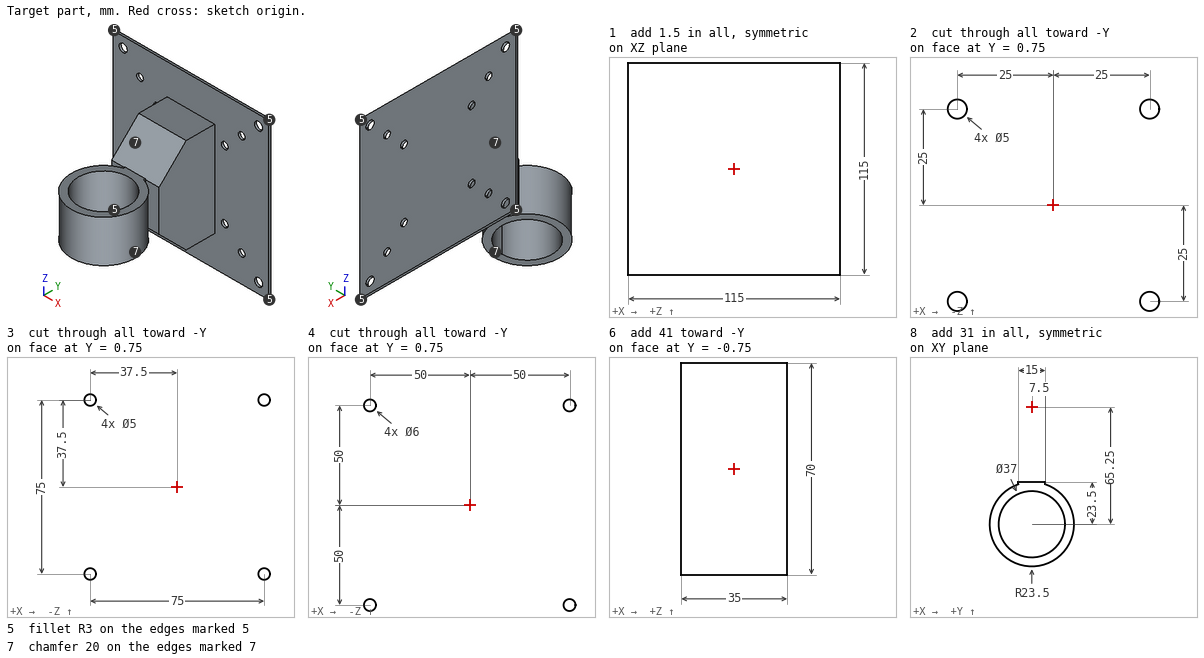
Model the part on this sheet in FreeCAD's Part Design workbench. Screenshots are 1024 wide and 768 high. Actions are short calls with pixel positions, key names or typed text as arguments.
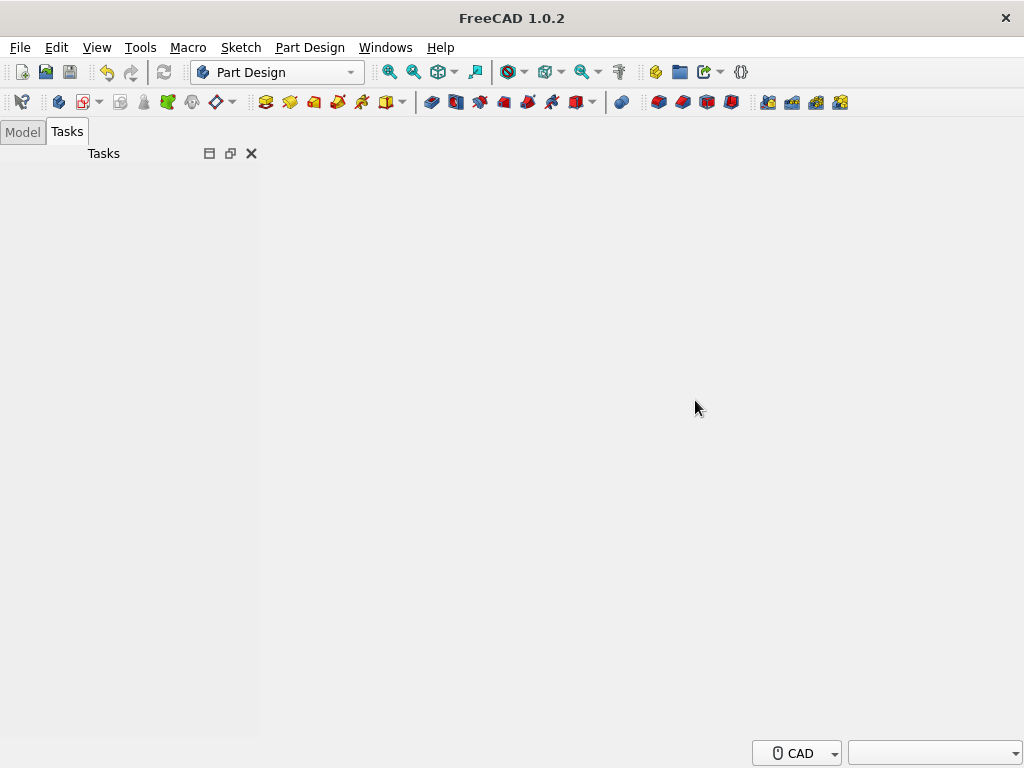
click(22, 72)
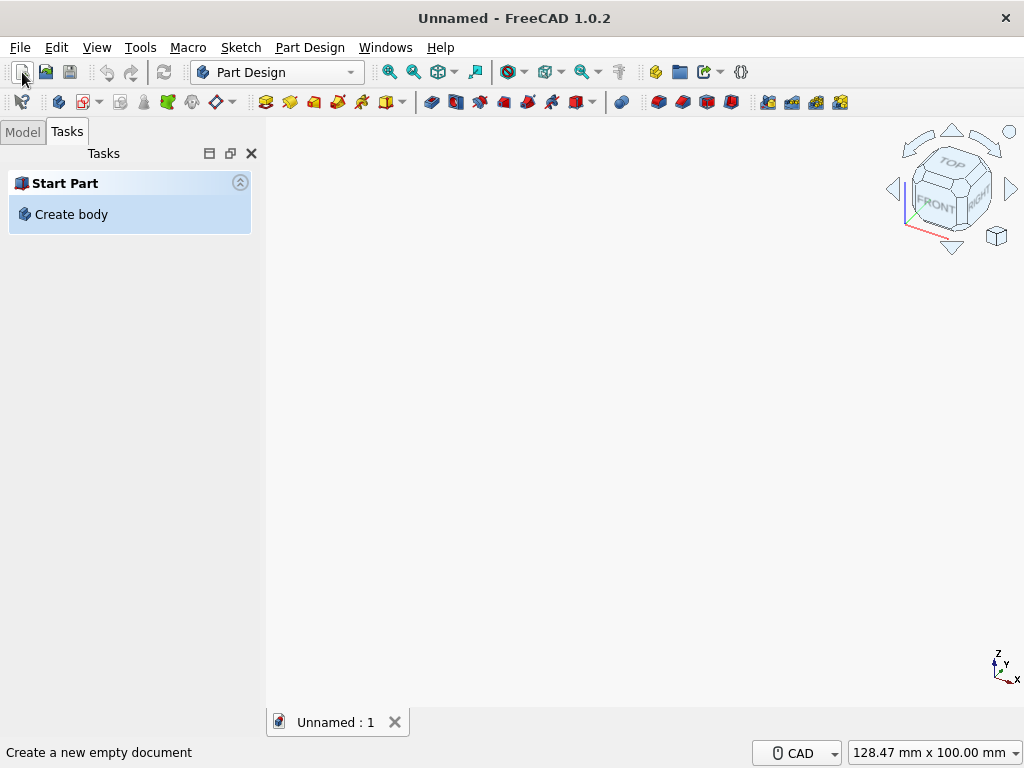
click(84, 102)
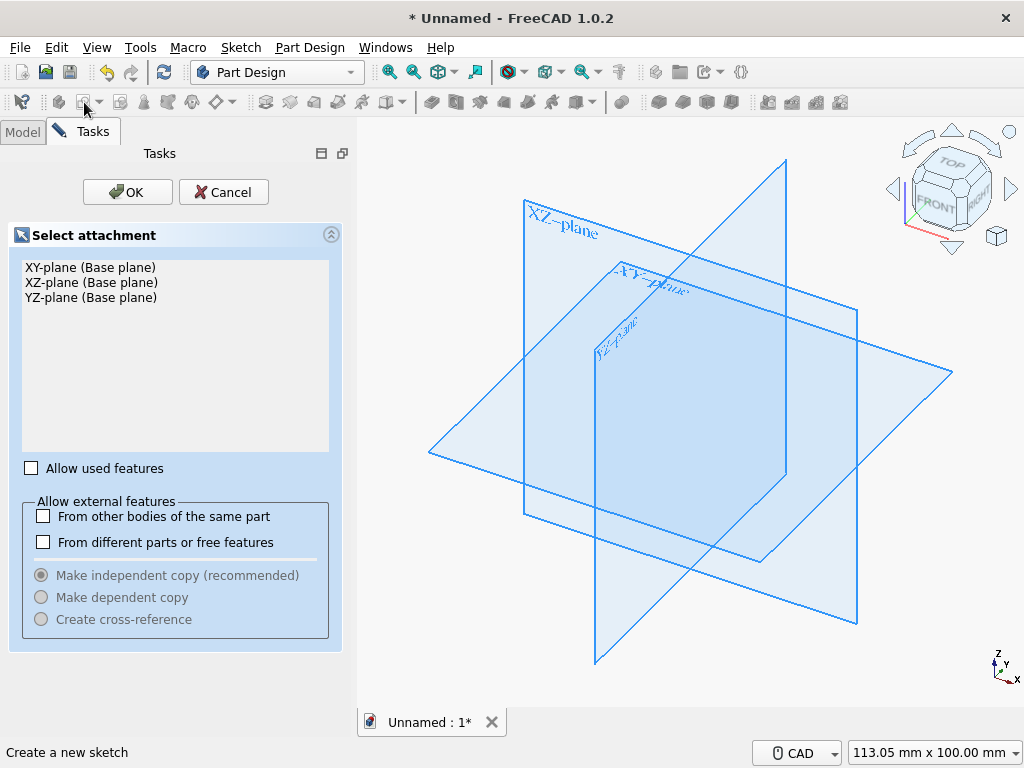
click(82, 282)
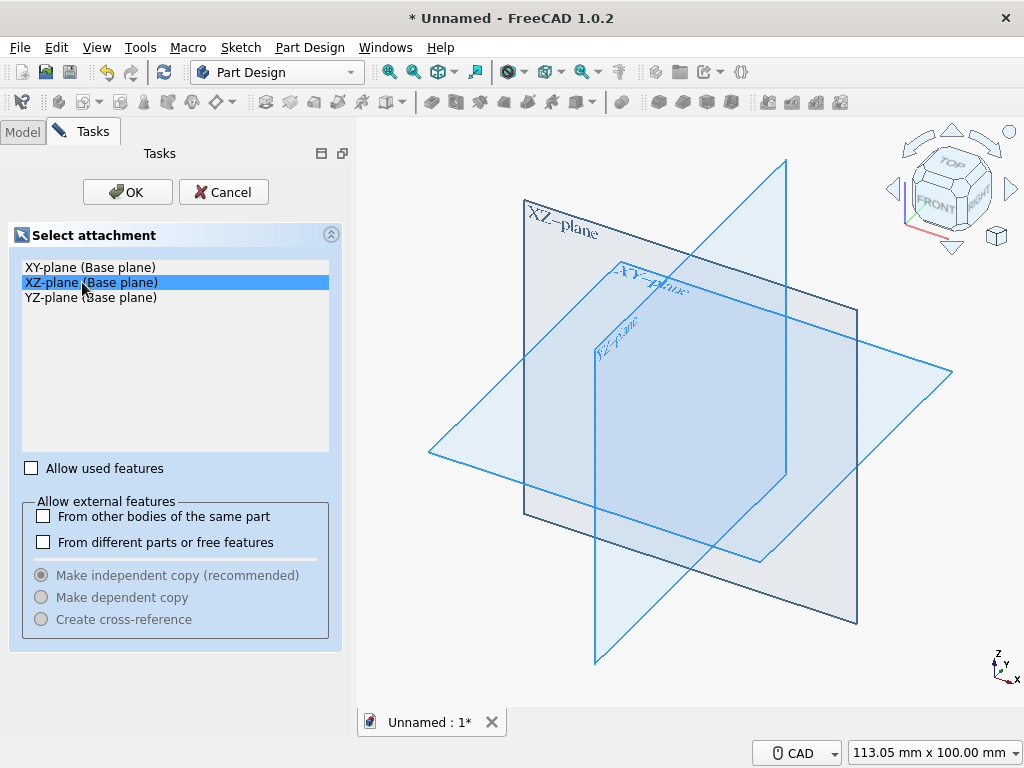
click(128, 192)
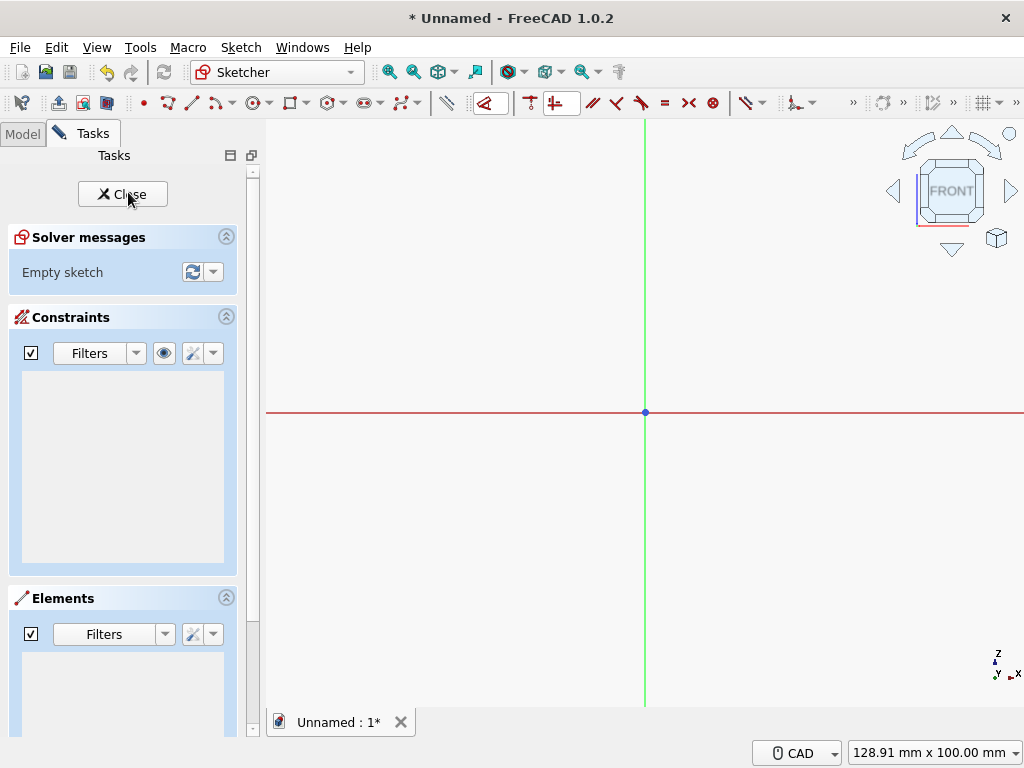
scroll(493, 413, down, 3)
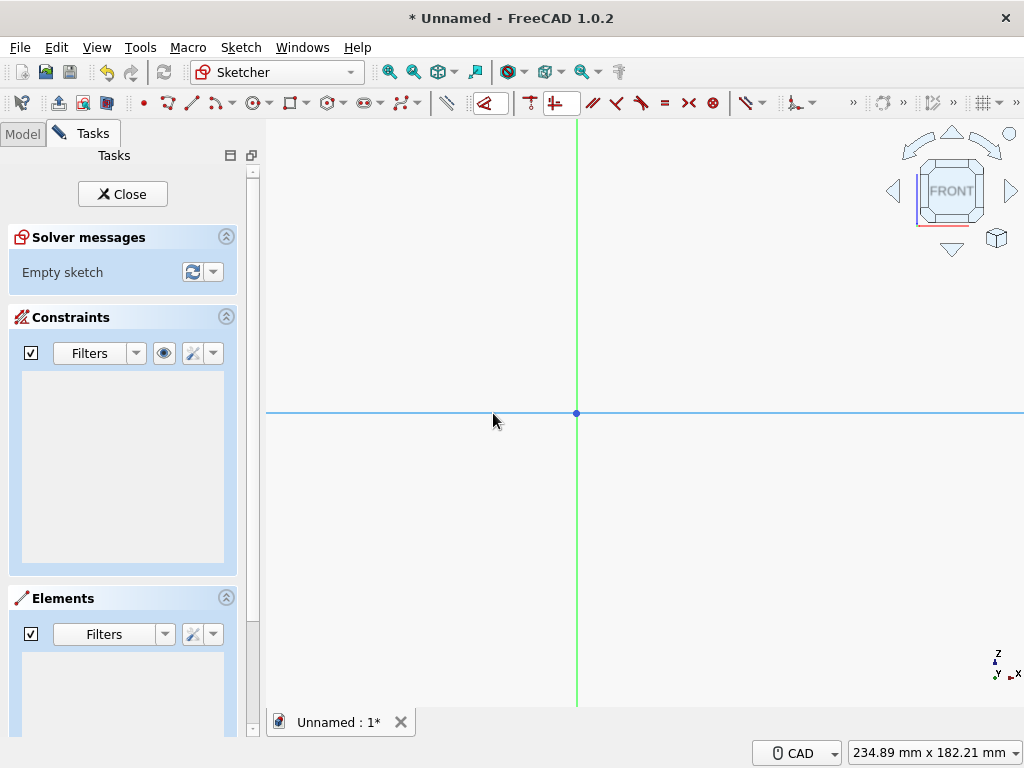
key(g)
key(v)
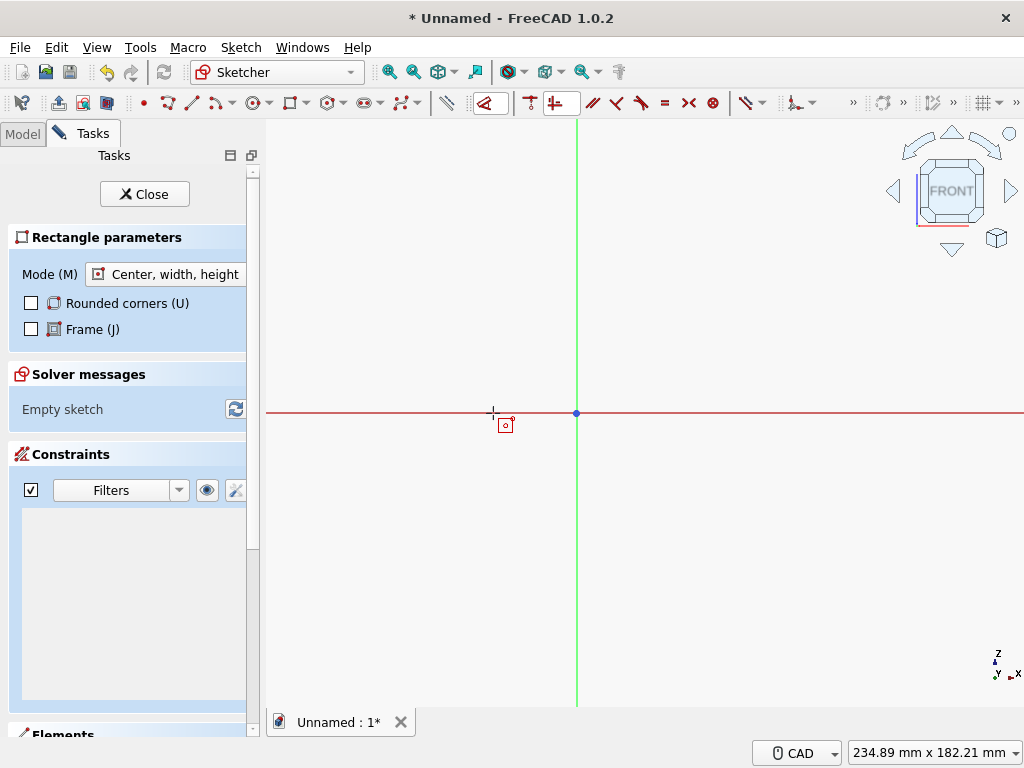
click(577, 413)
click(762, 228)
key(Escape)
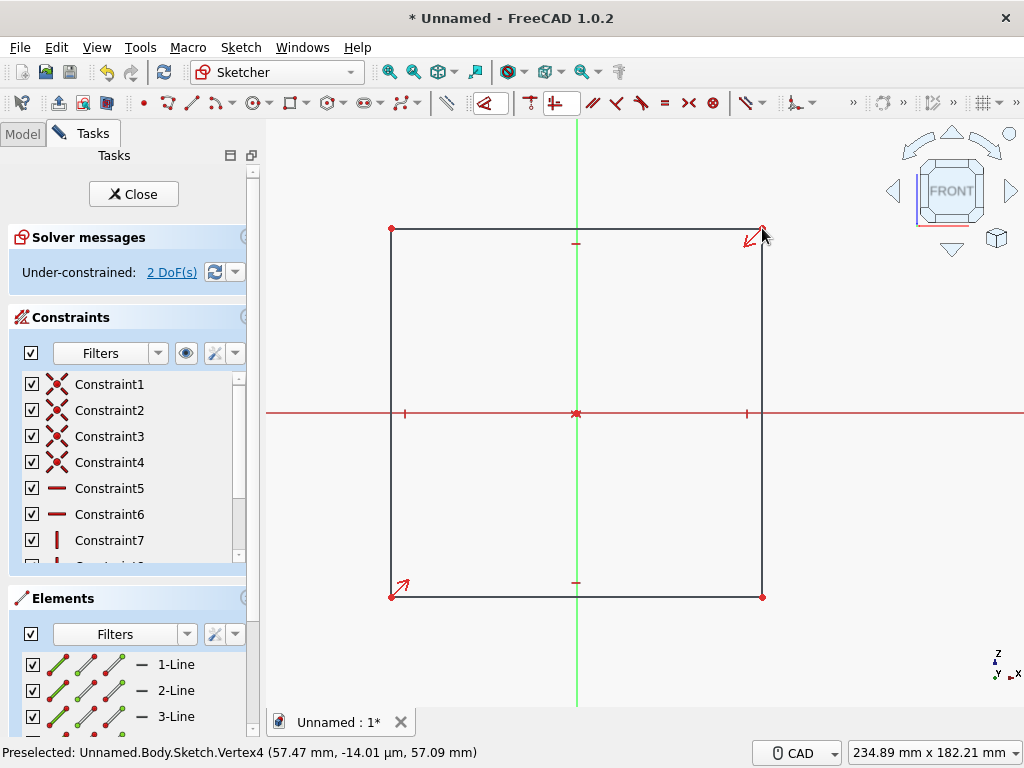
key(d)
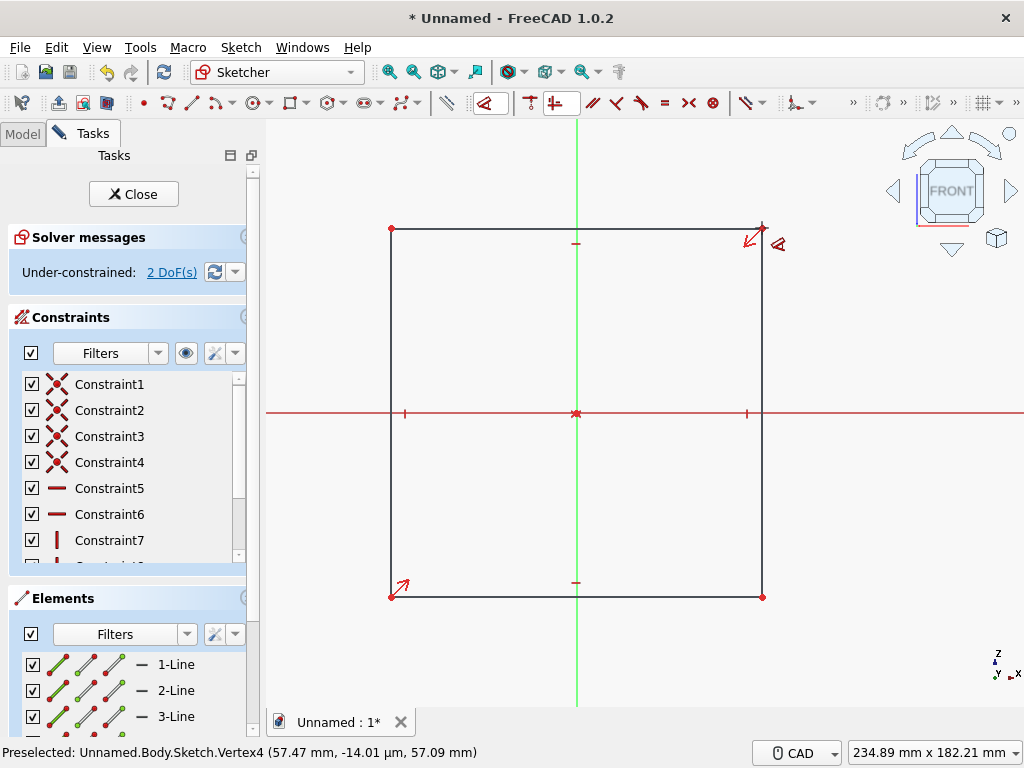
click(502, 597)
click(491, 631)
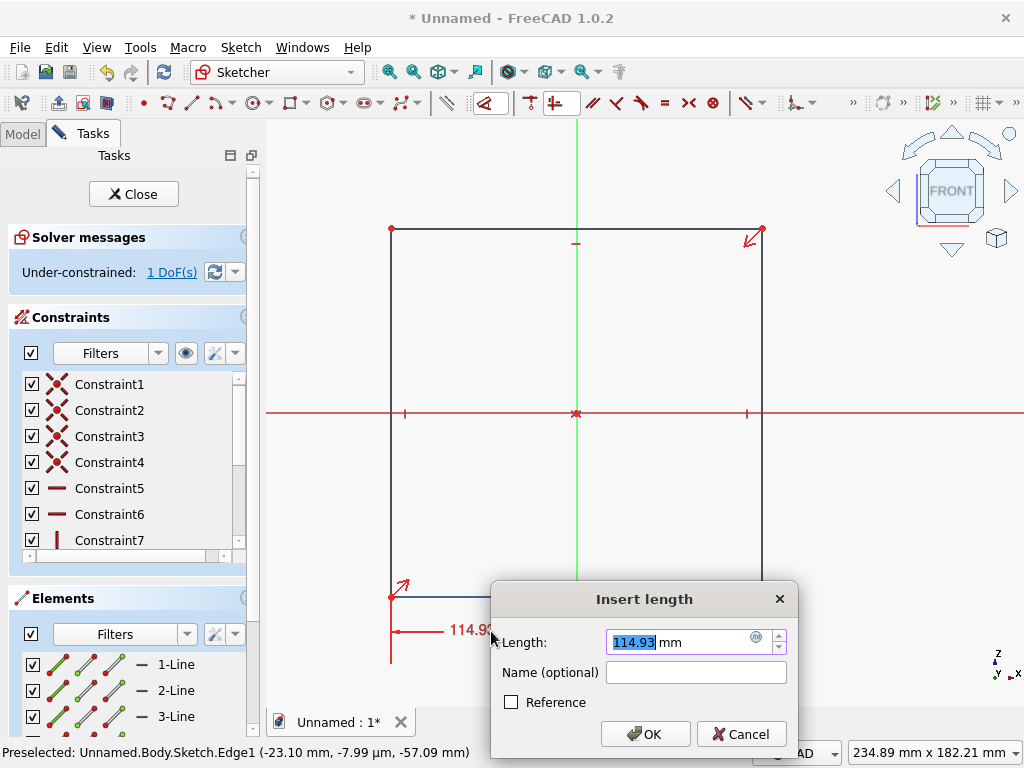
text(115)
key(Return)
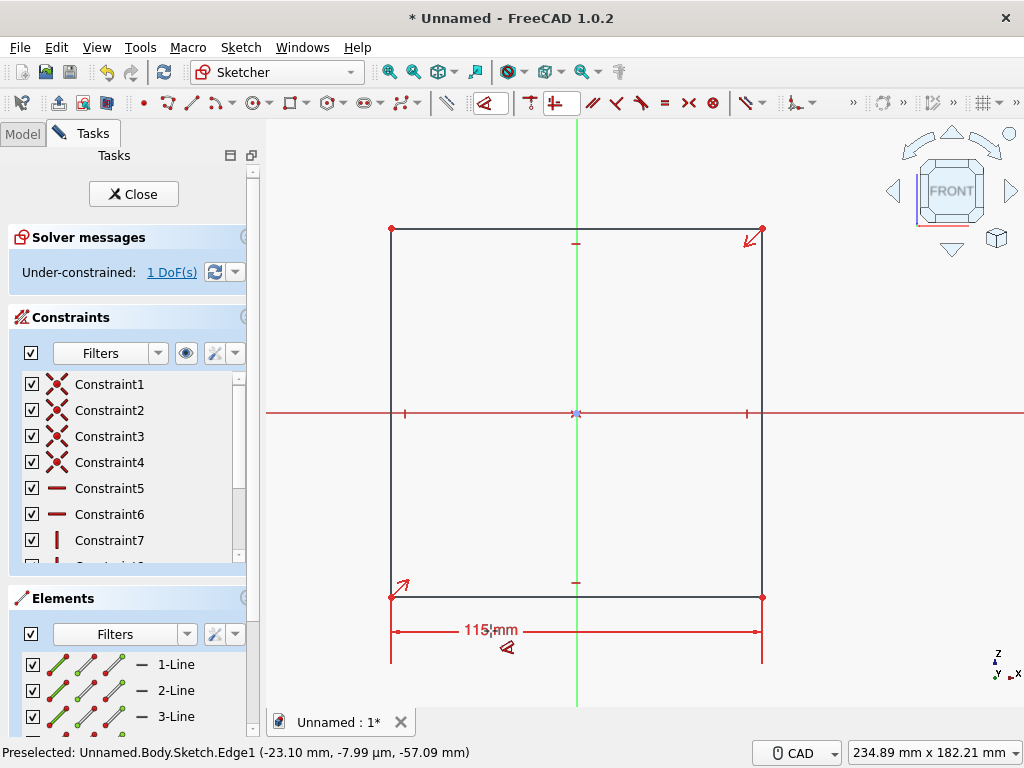
click(762, 487)
click(796, 328)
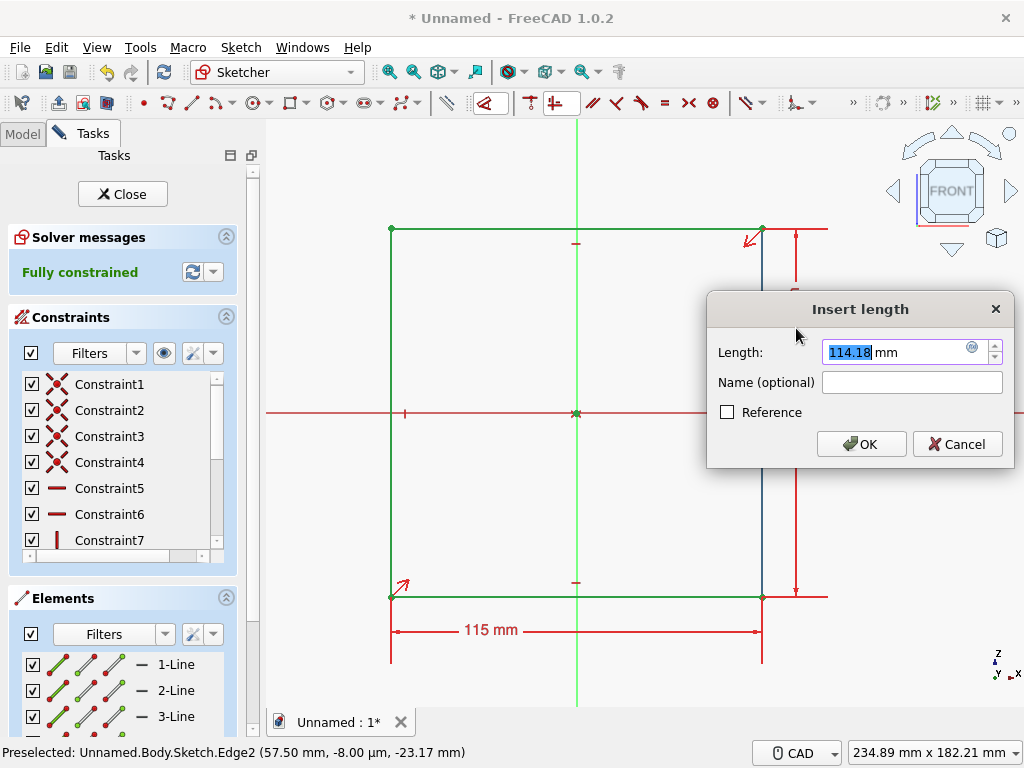
text(115)
key(Return)
key(Escape)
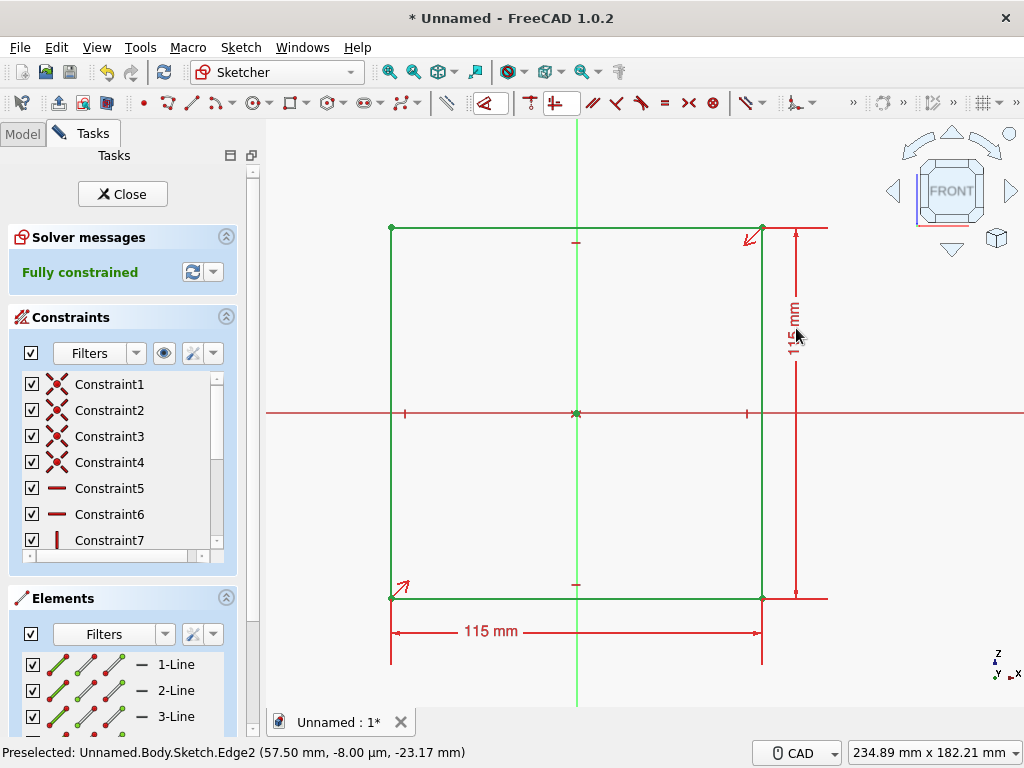
click(123, 194)